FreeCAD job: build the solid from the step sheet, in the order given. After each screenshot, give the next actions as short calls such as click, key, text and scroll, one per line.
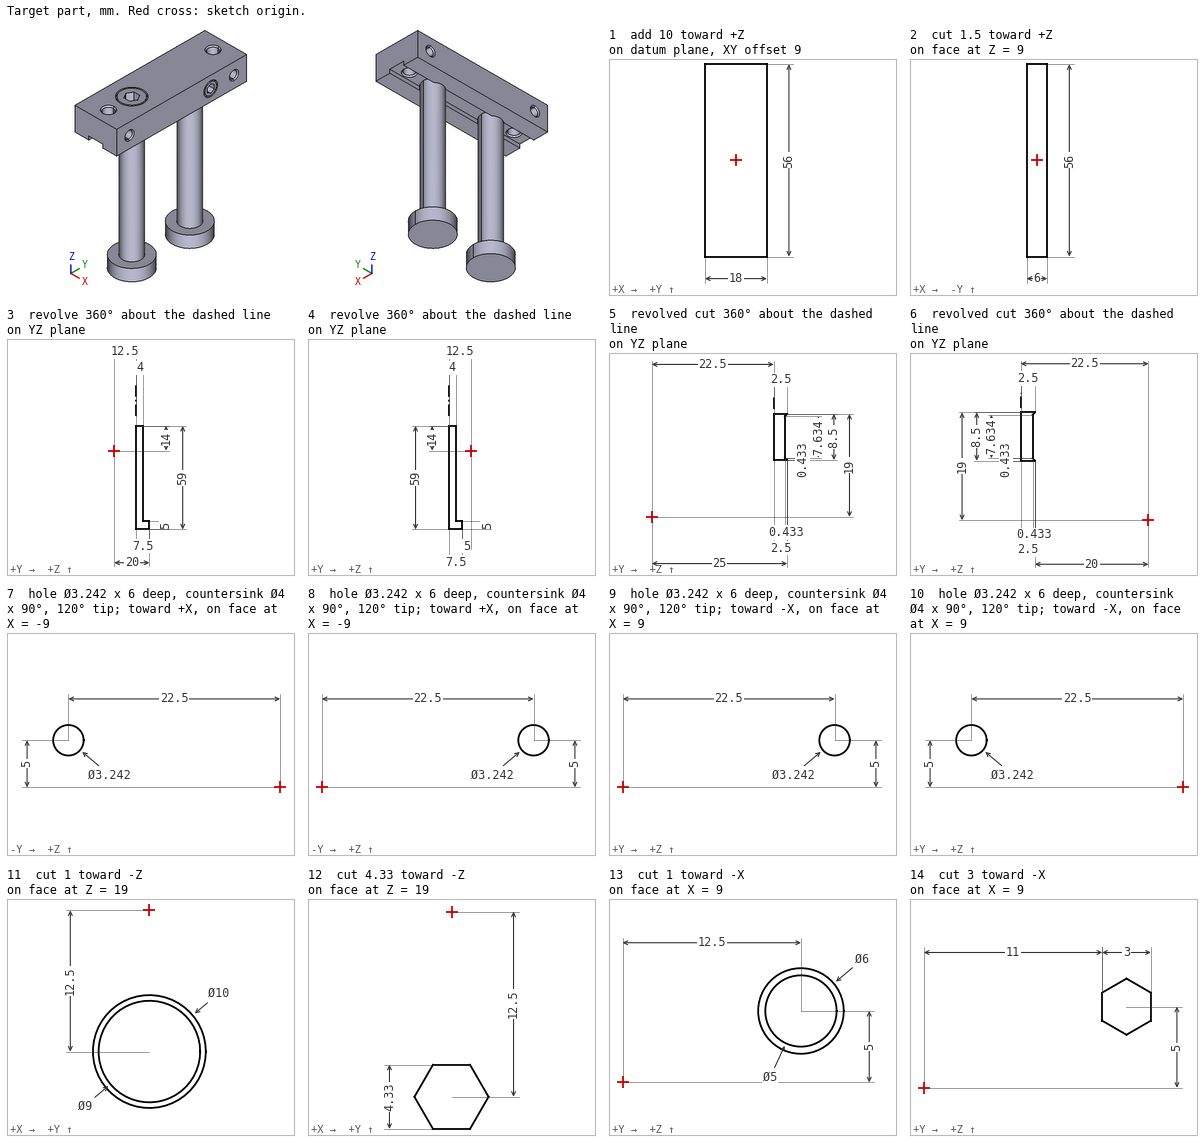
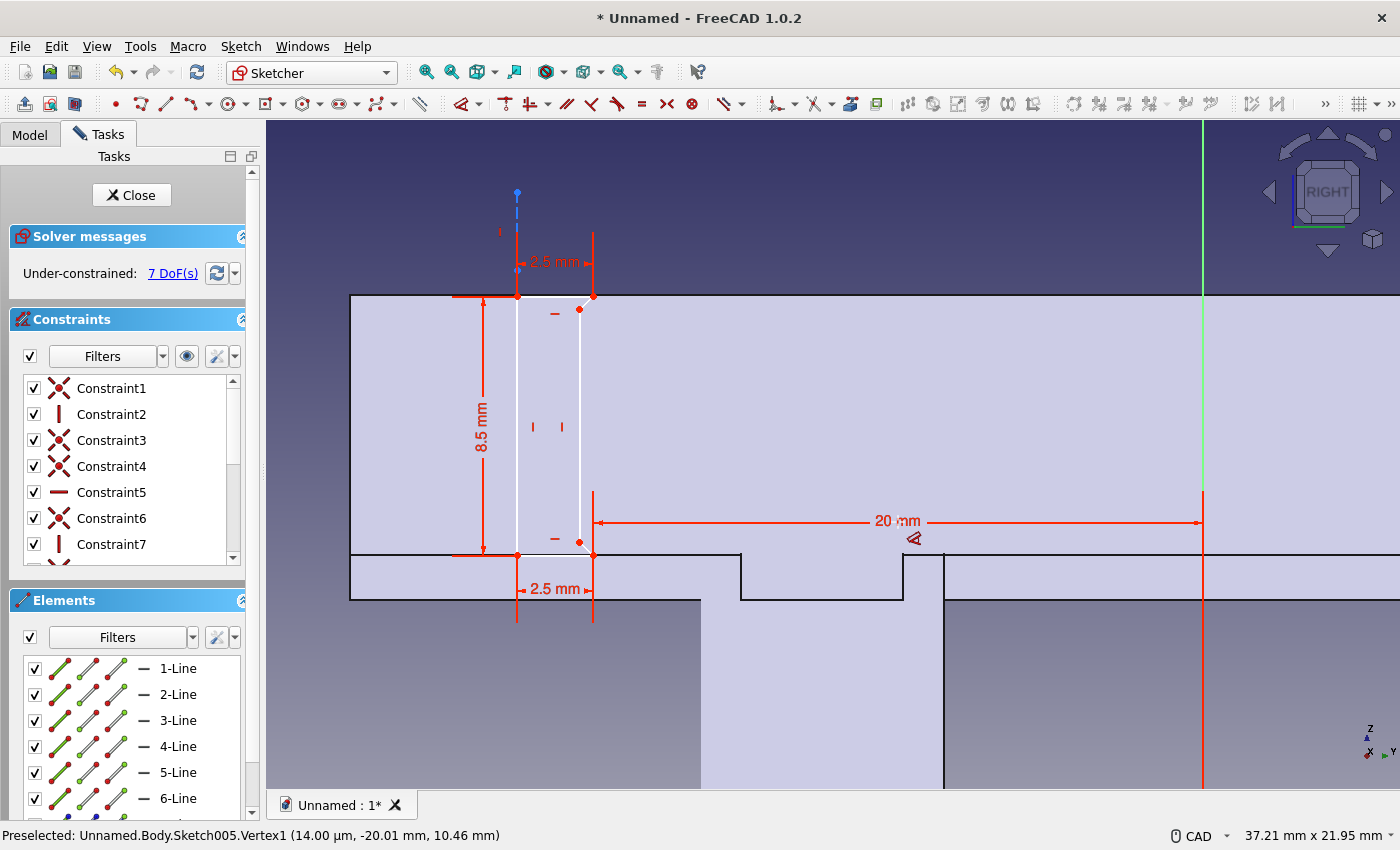
click(593, 297)
click(559, 529)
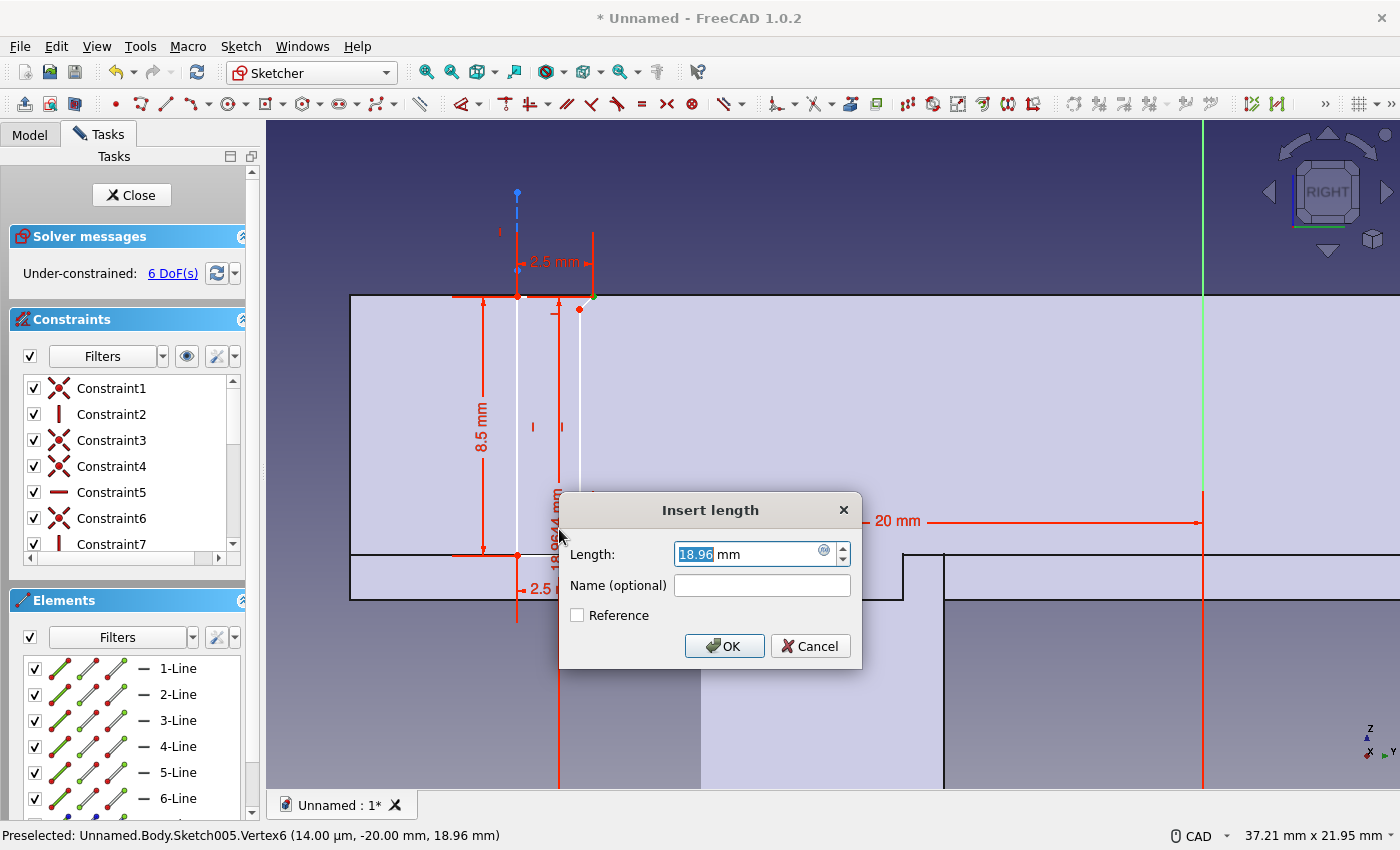
text(19)
key(Return)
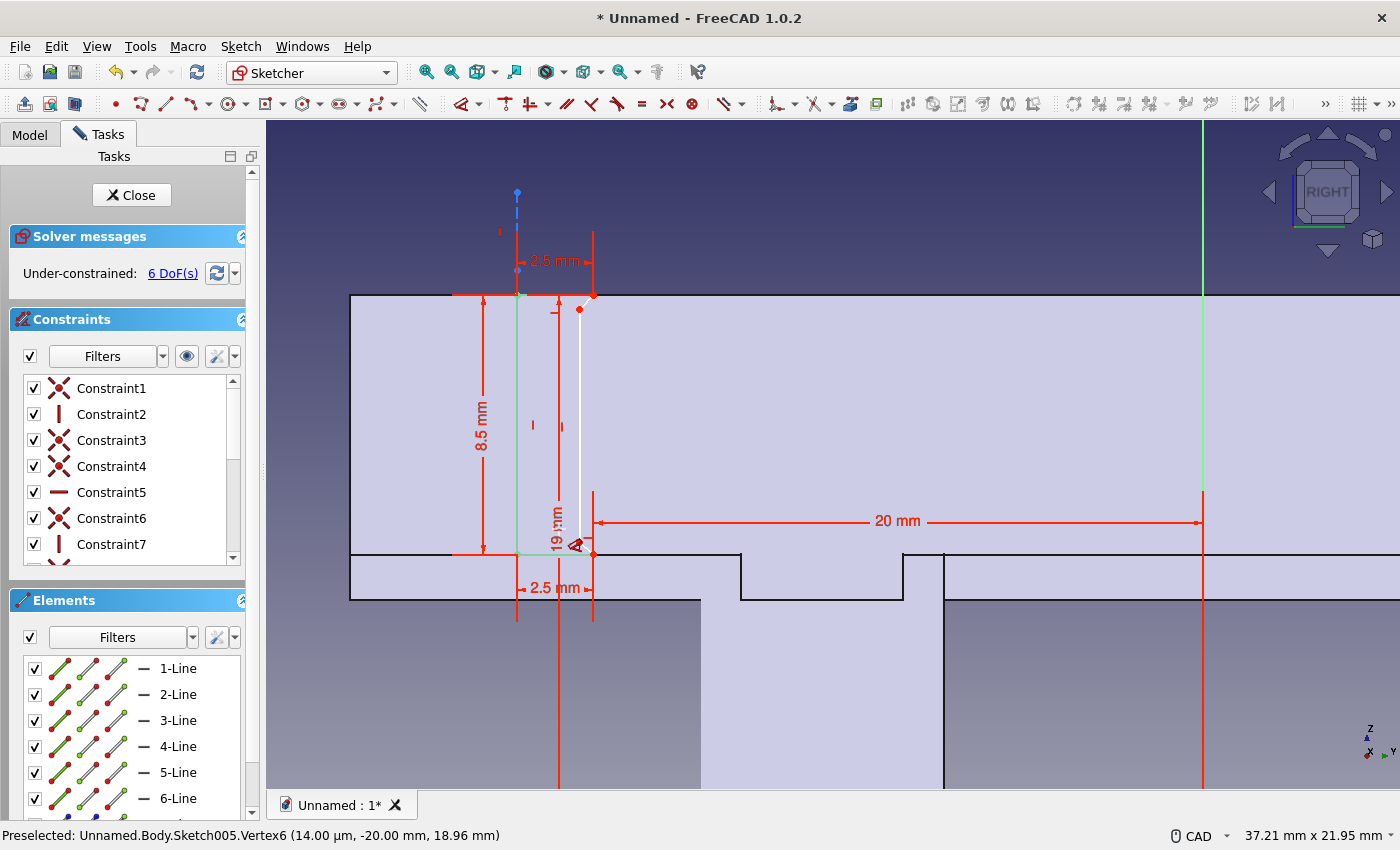
click(580, 473)
click(546, 372)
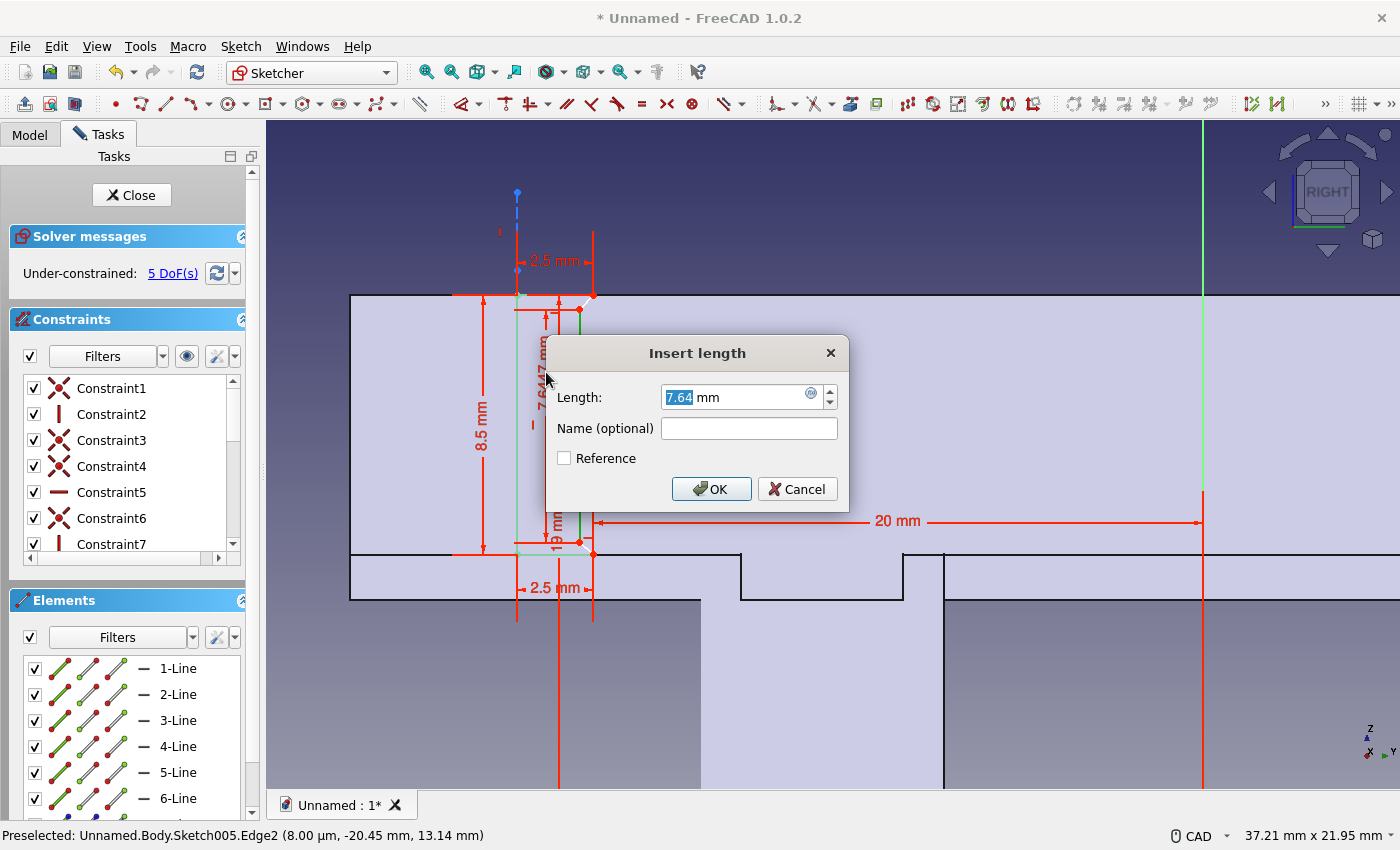
text(7.634)
key(Return)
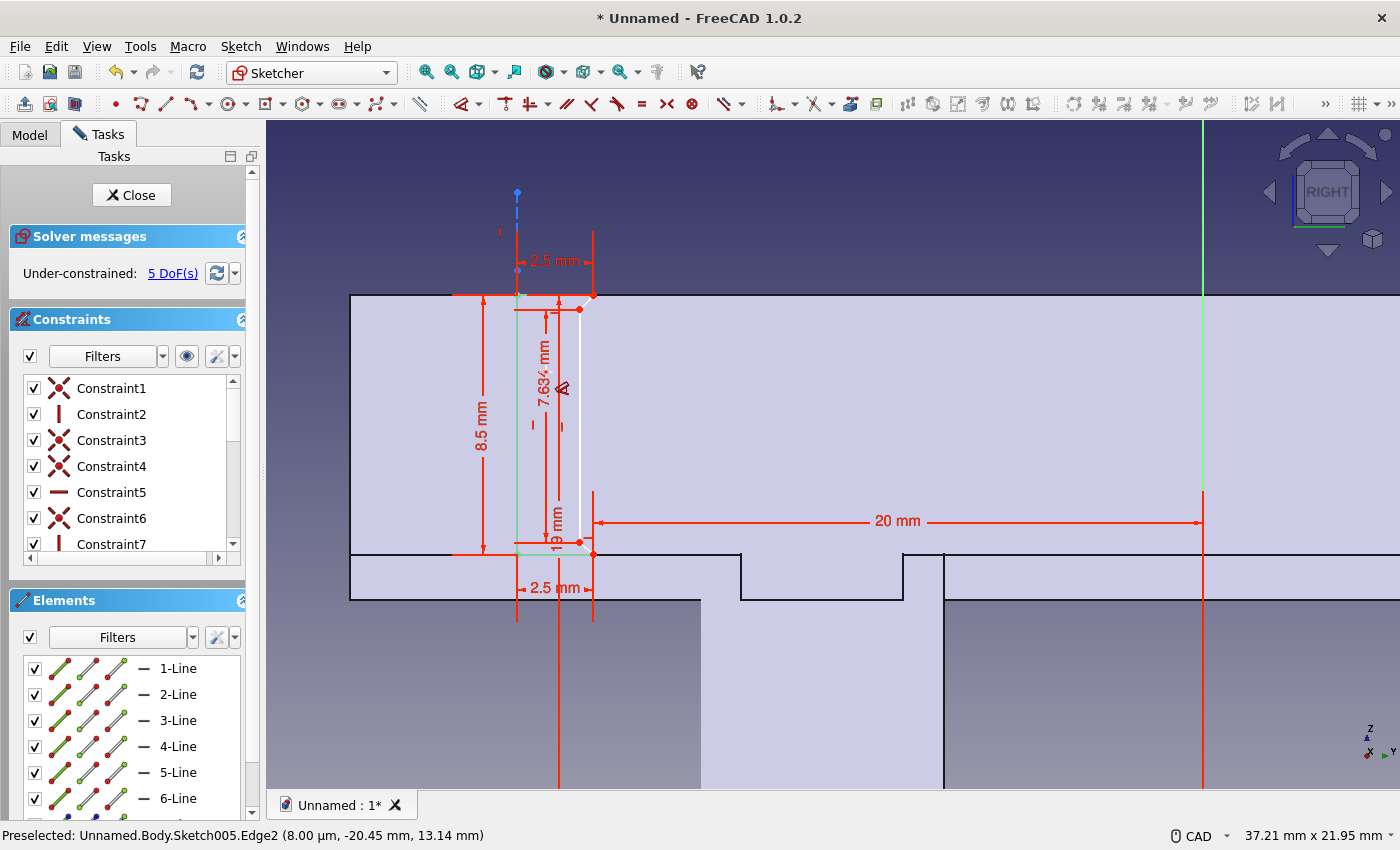
click(517, 271)
click(860, 237)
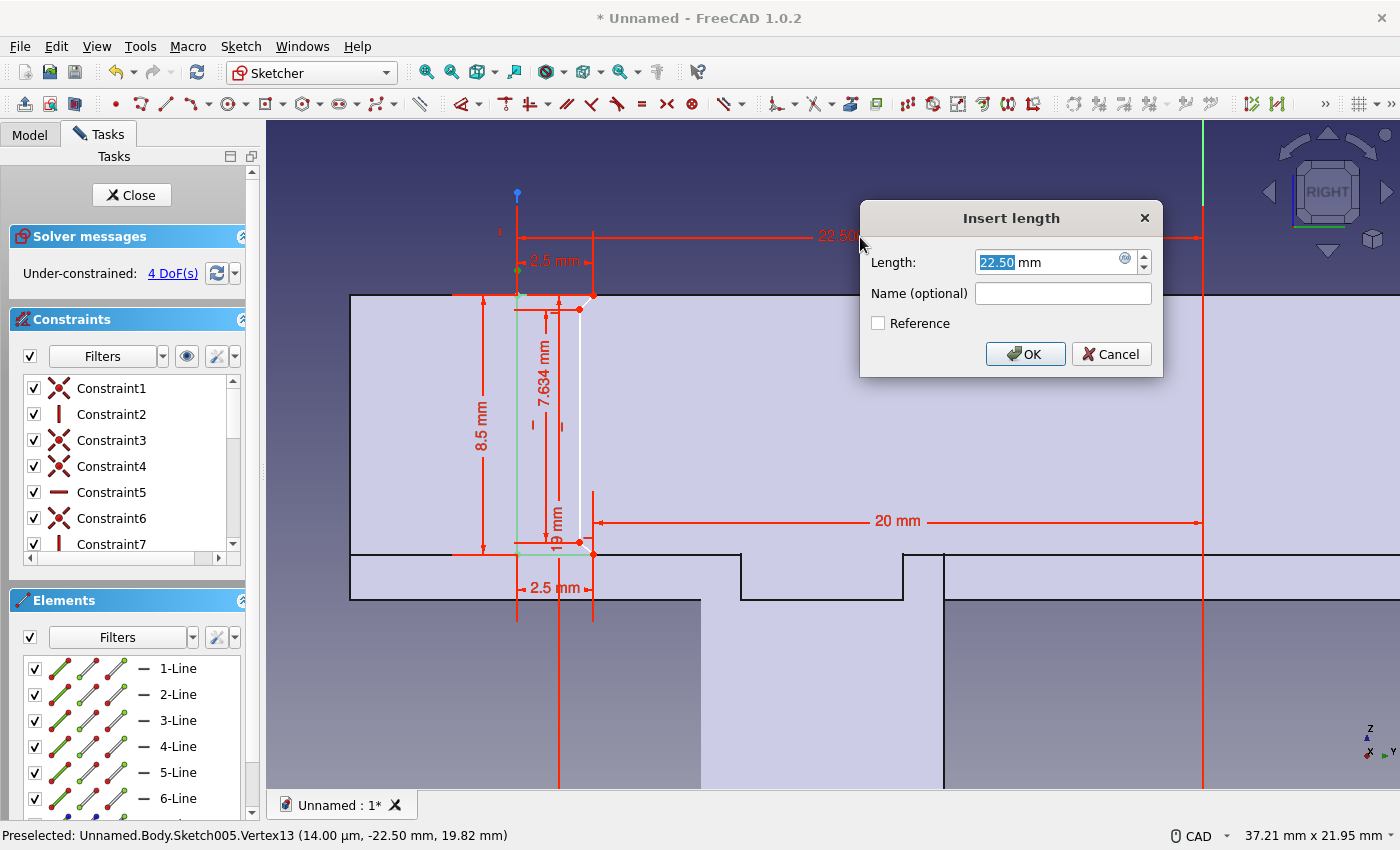
text(22.5)
key(Return)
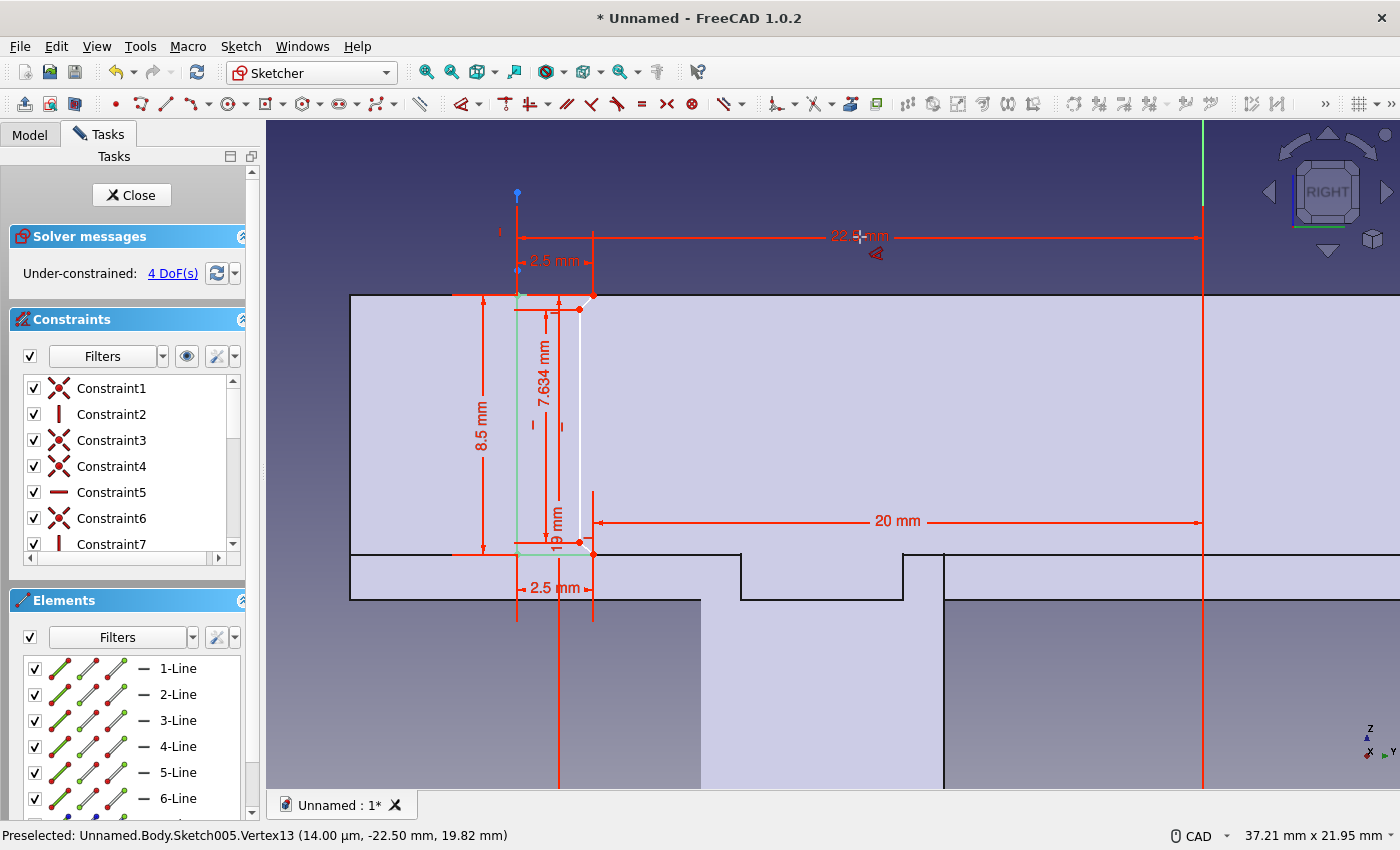
scroll(585, 547, up, 6)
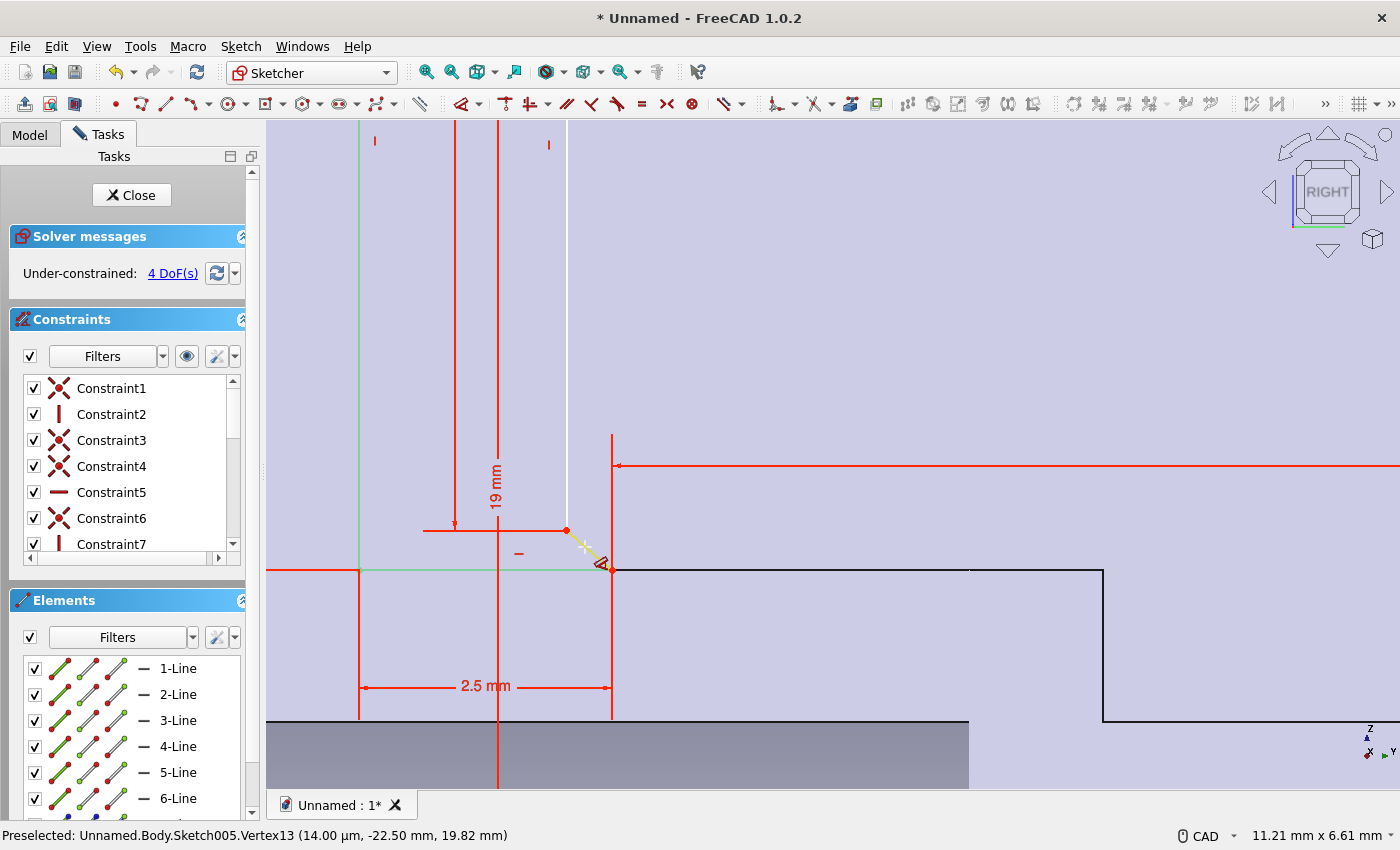
click(585, 547)
click(589, 604)